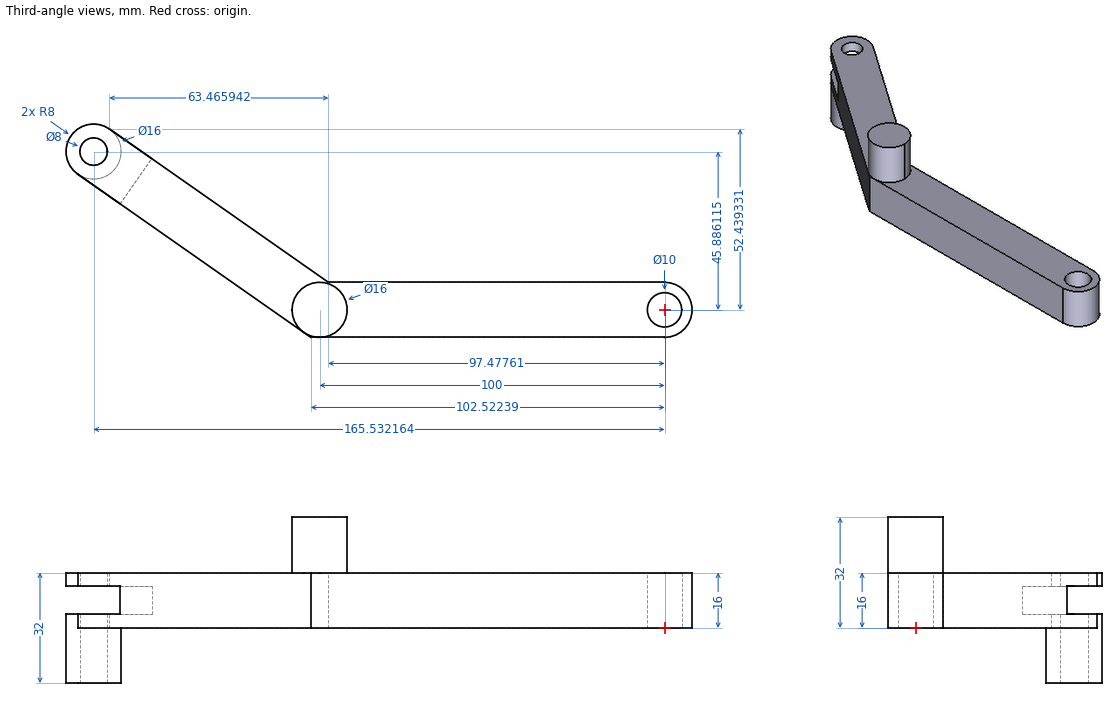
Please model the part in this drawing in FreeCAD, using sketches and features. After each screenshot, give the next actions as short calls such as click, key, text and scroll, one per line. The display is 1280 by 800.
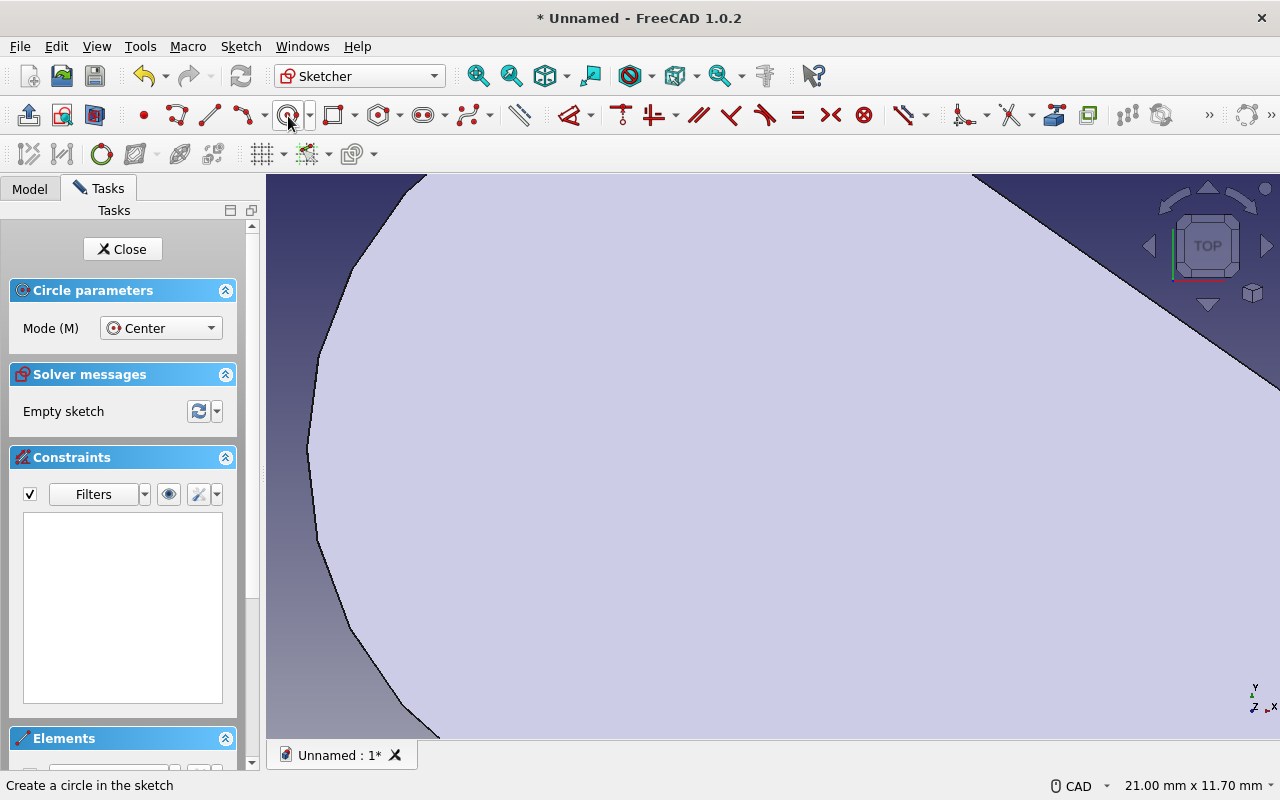
click(693, 451)
click(830, 314)
key(Escape)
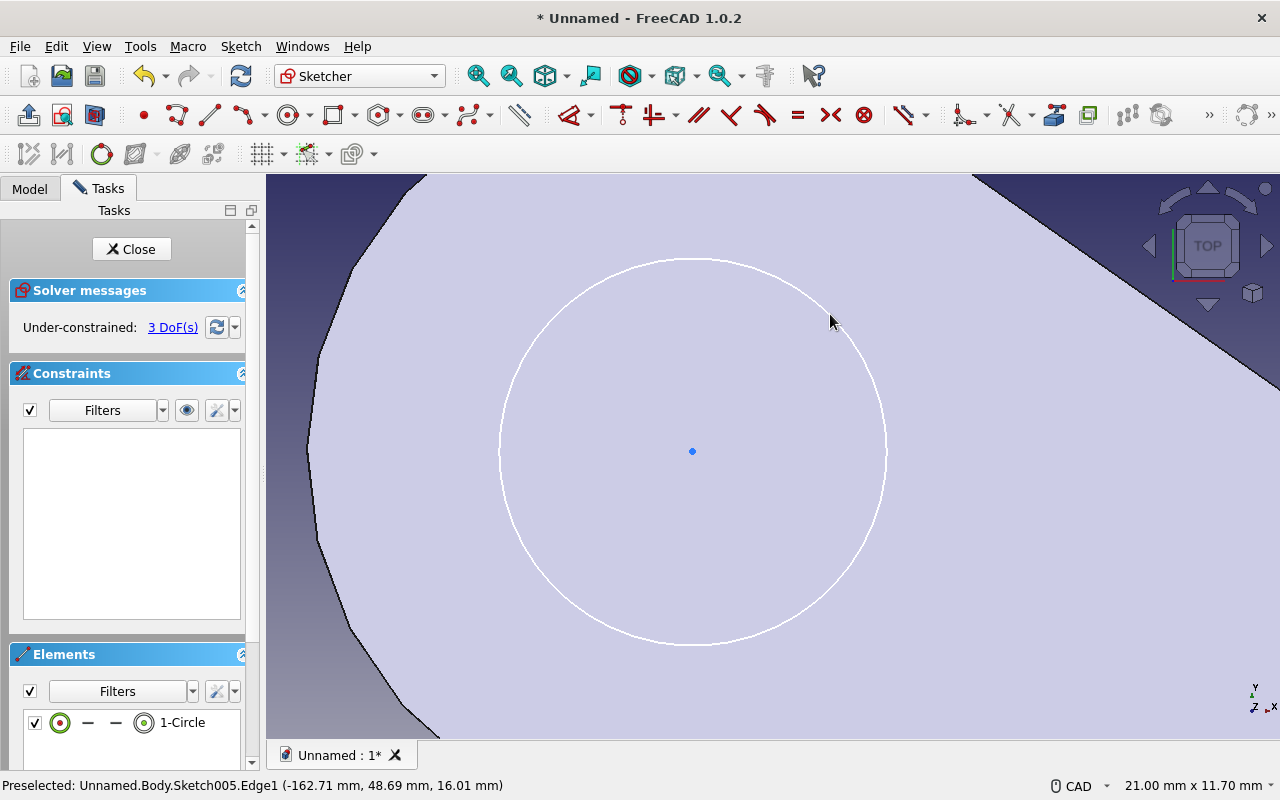
click(568, 116)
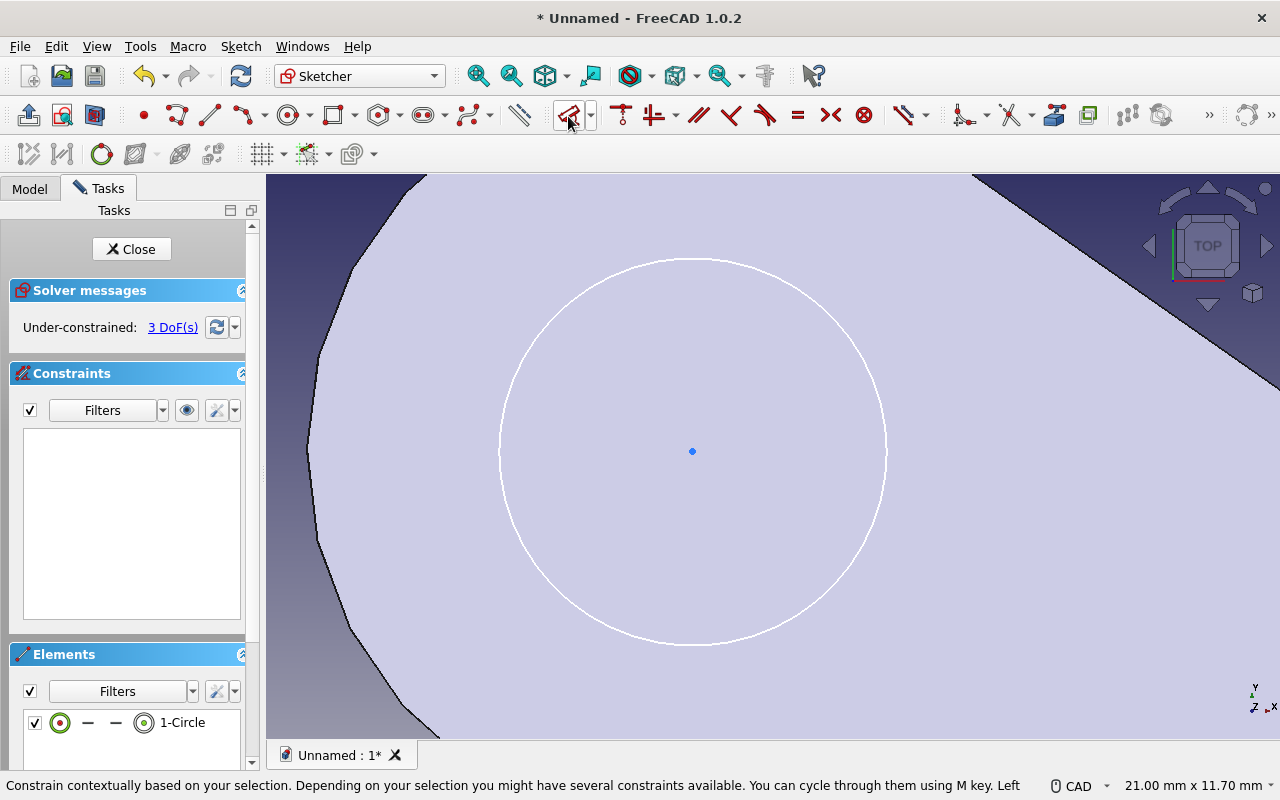
click(830, 315)
click(853, 292)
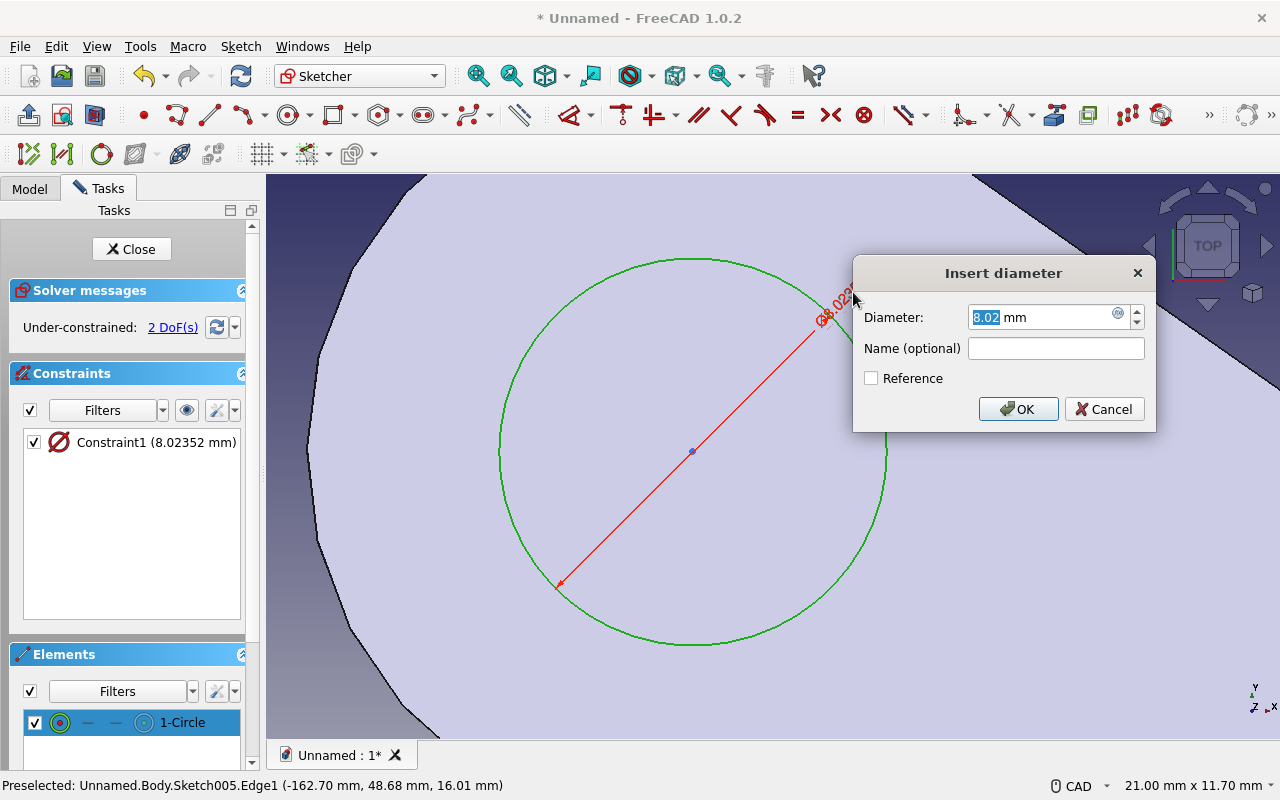
text(8)
key(Return)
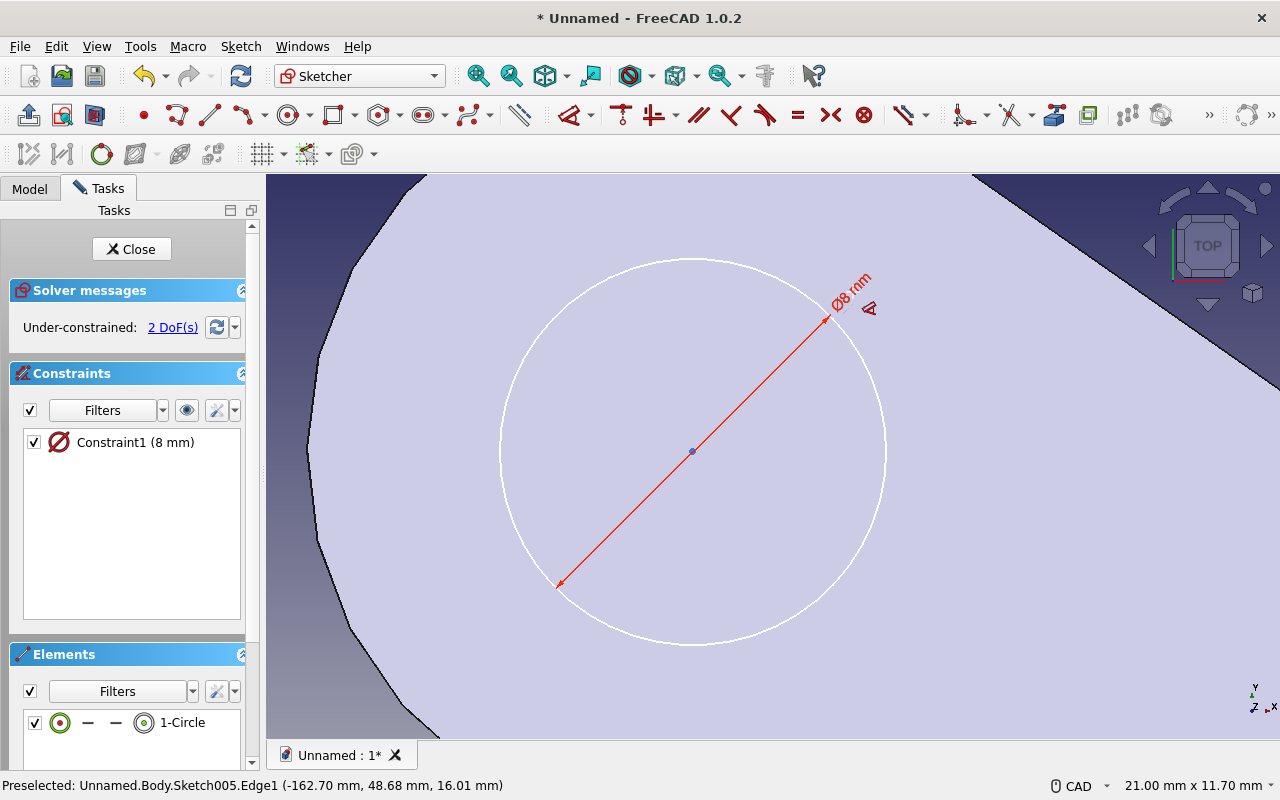
click(693, 452)
click(659, 582)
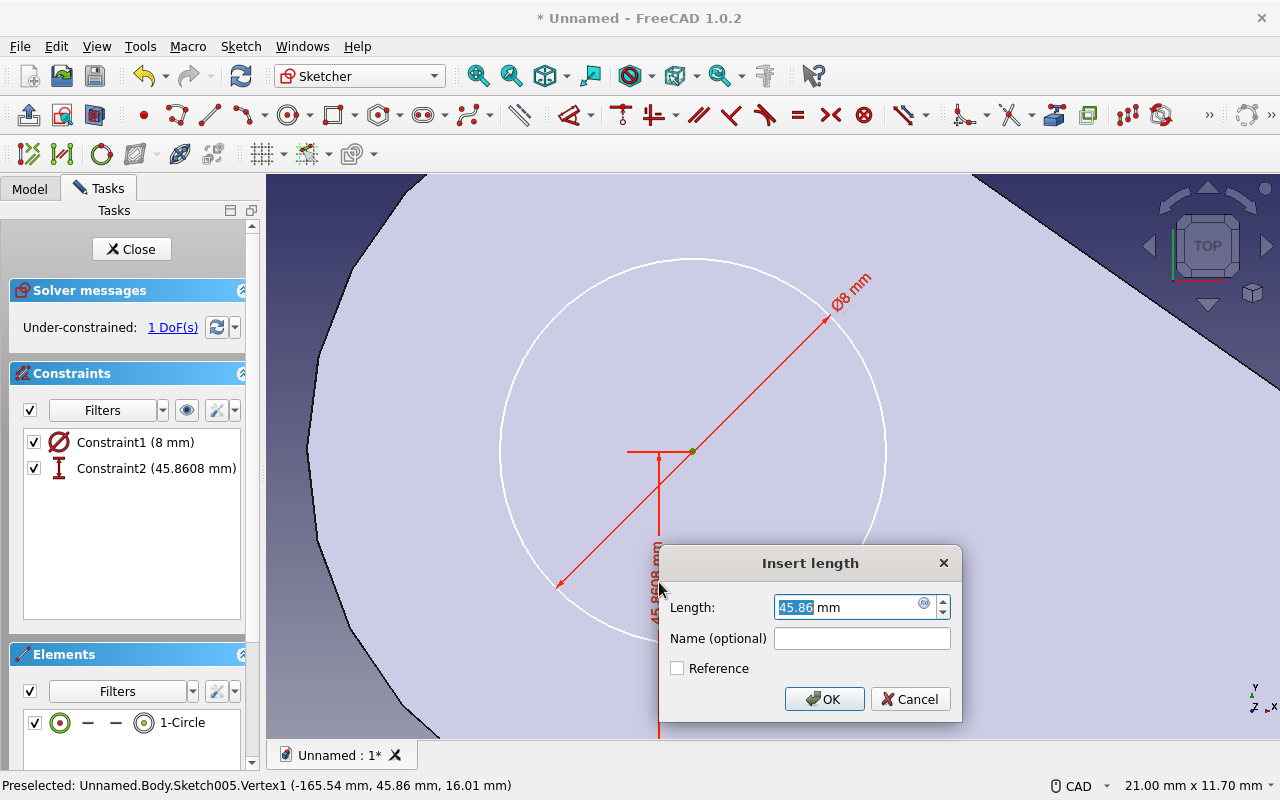
text(45.886115)
key(Return)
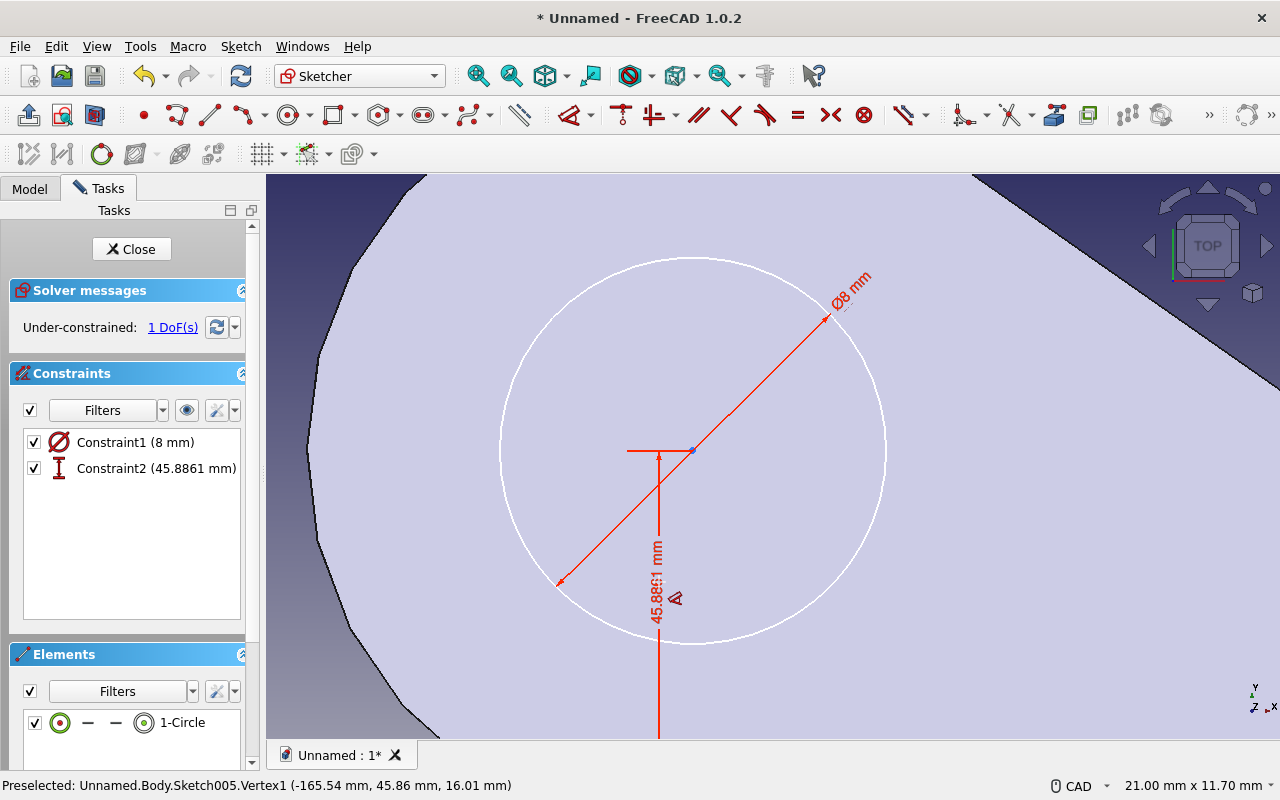
click(693, 451)
click(904, 417)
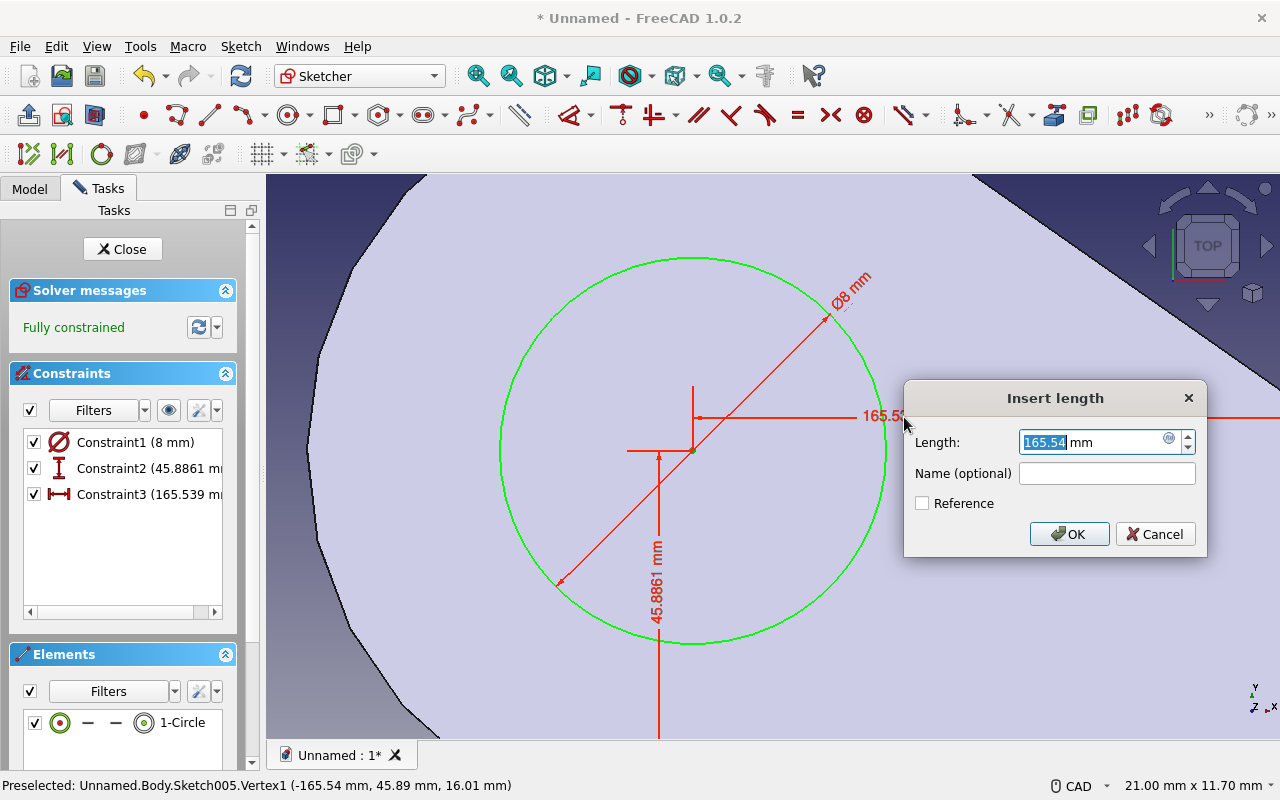
text(165.532164)
key(Return)
key(Escape)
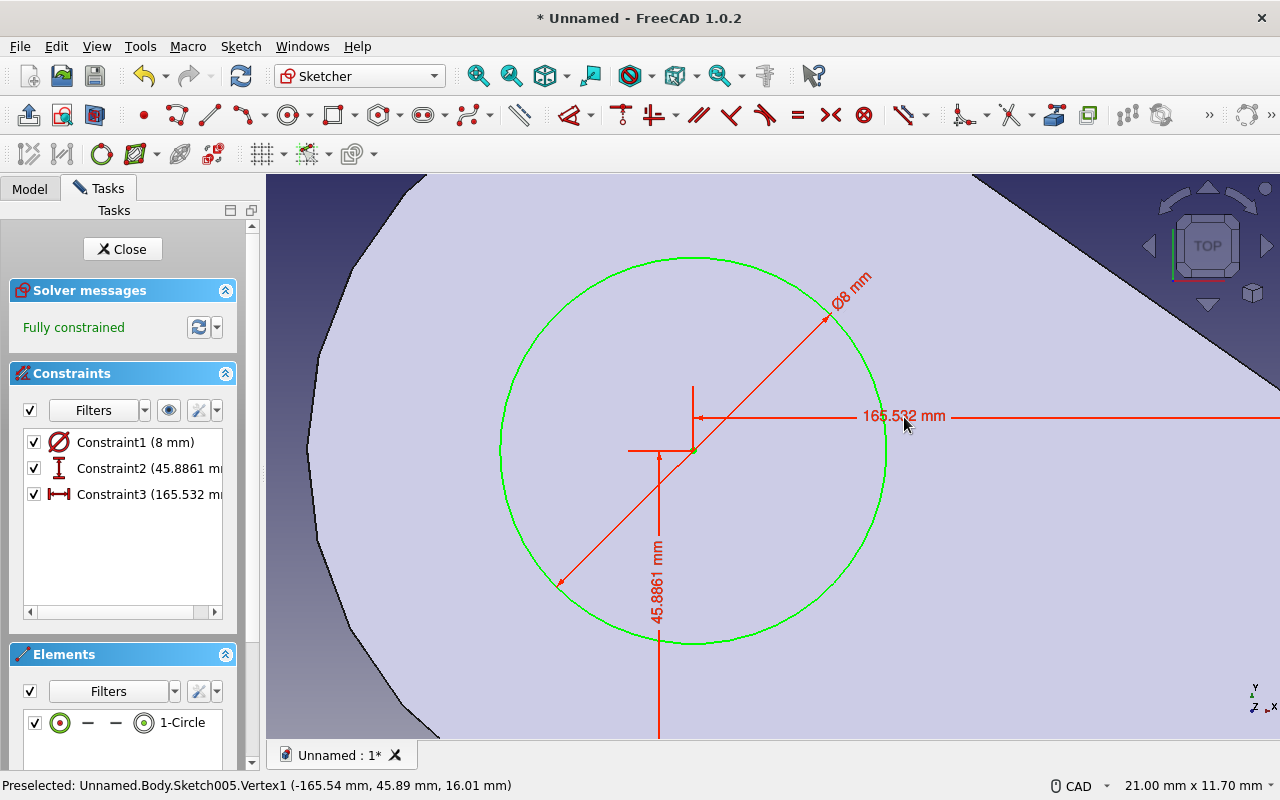
click(123, 249)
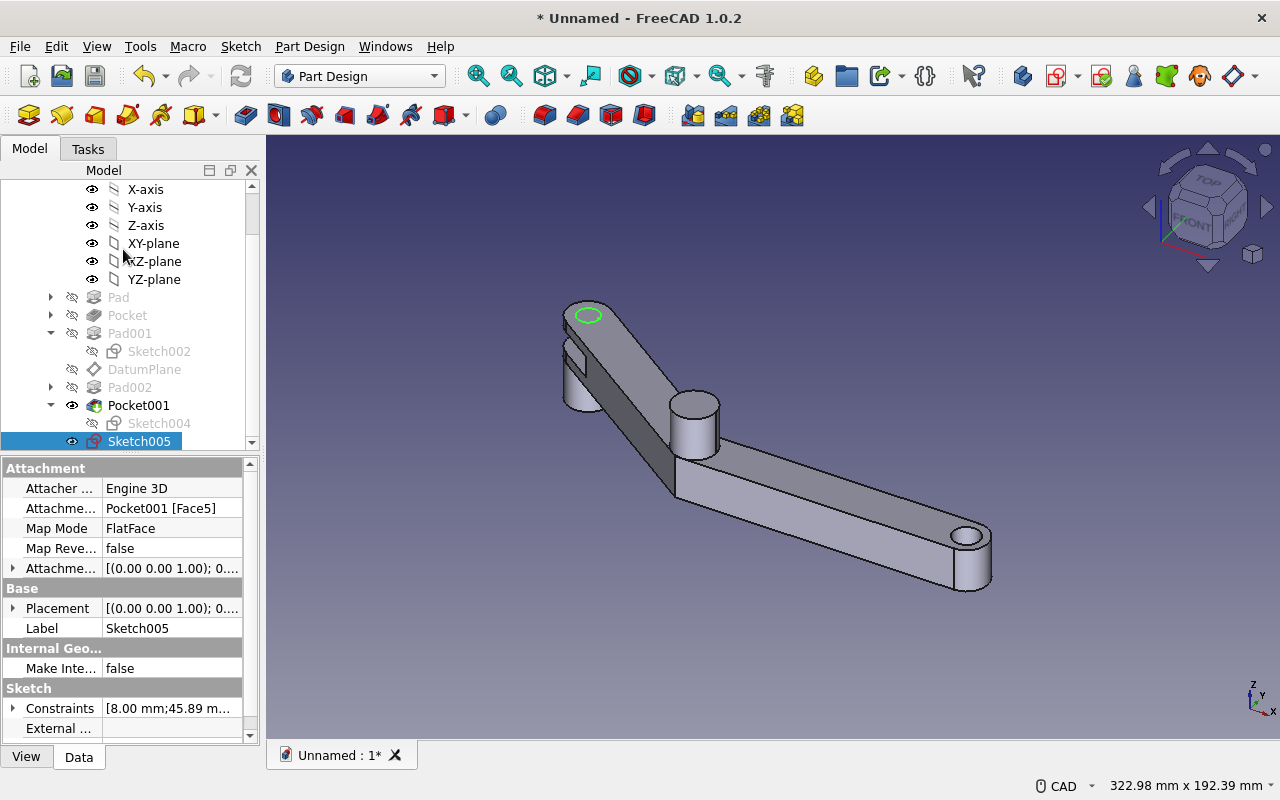
click(246, 116)